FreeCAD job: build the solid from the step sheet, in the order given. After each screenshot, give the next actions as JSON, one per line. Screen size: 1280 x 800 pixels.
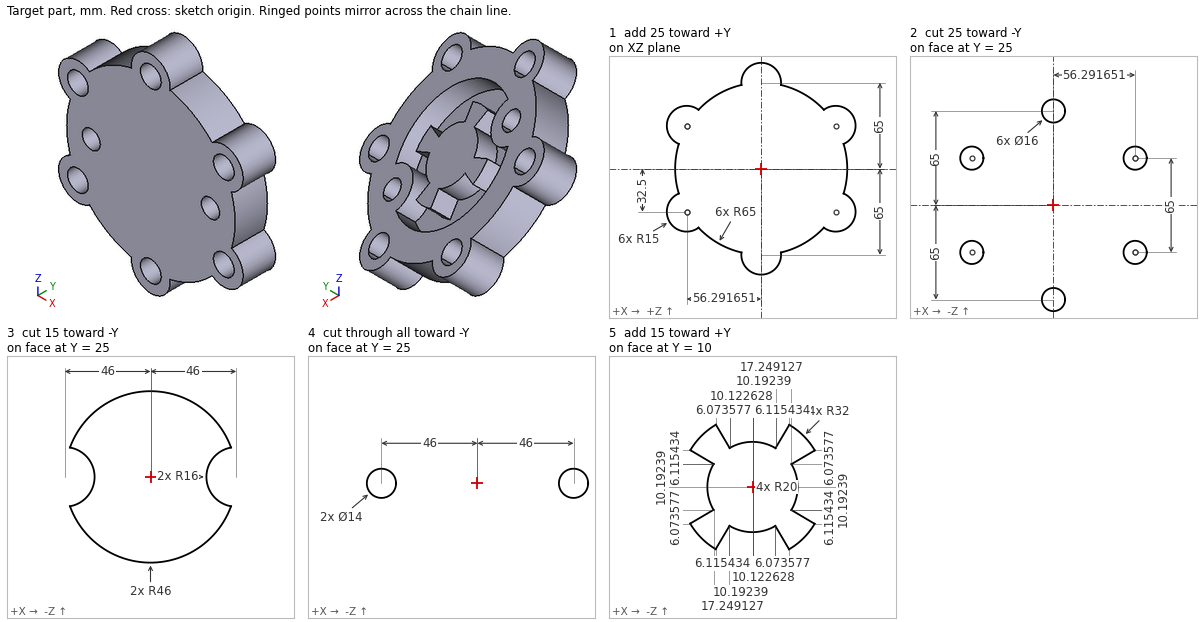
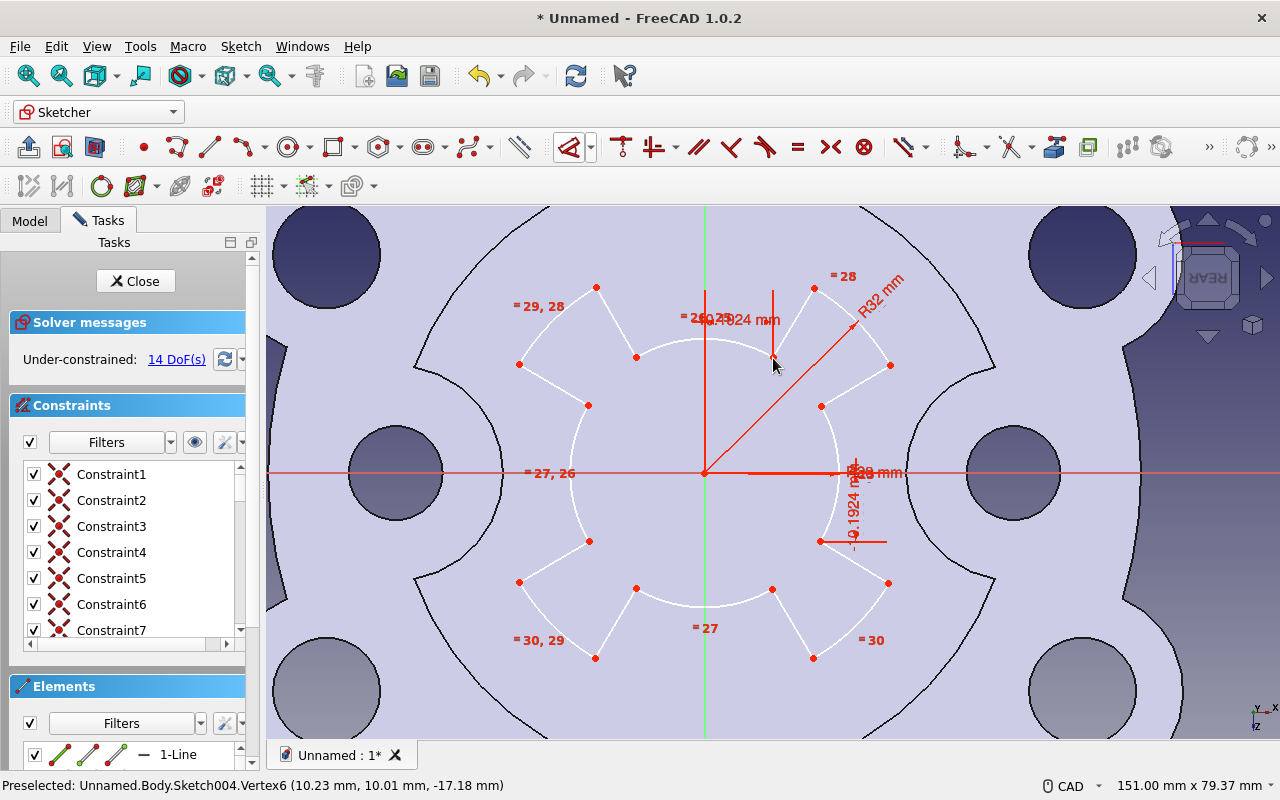
{"action": "left_click", "coordinate": [589, 406]}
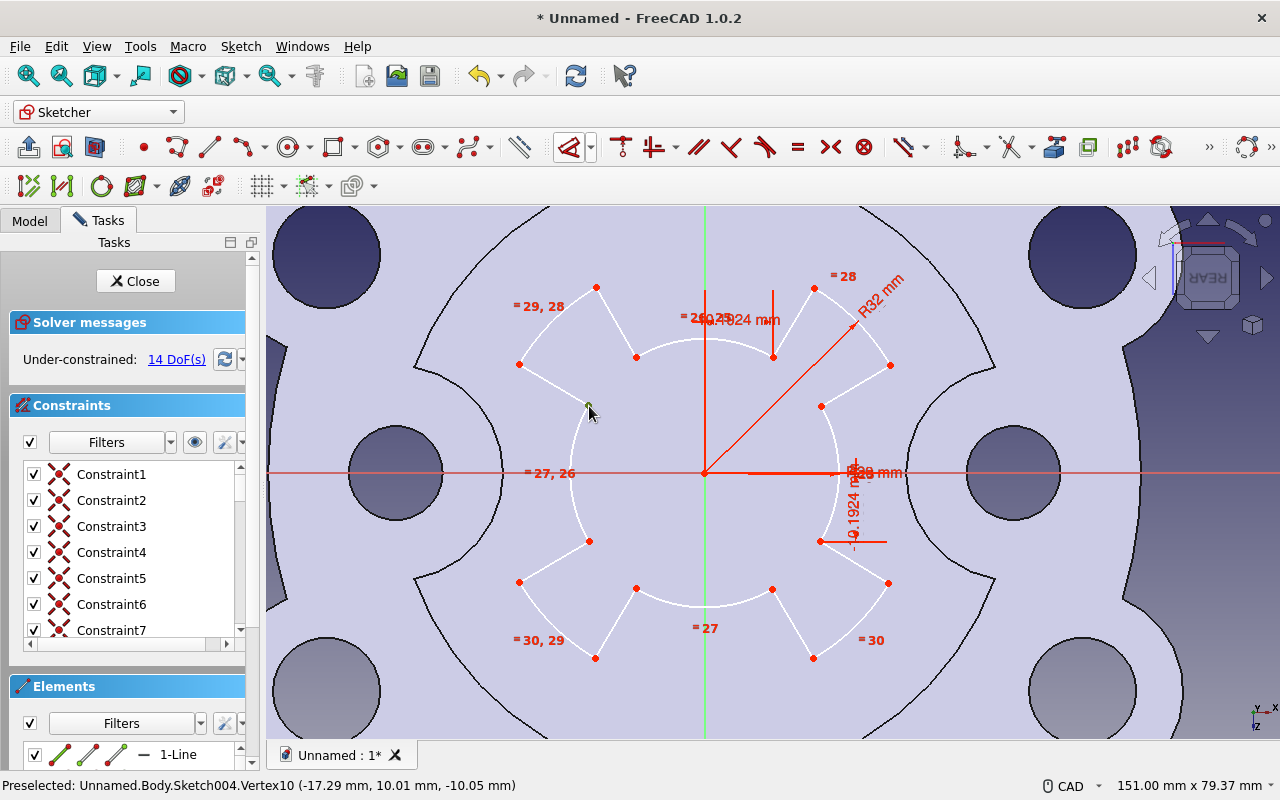
{"action": "left_click", "coordinate": [590, 148]}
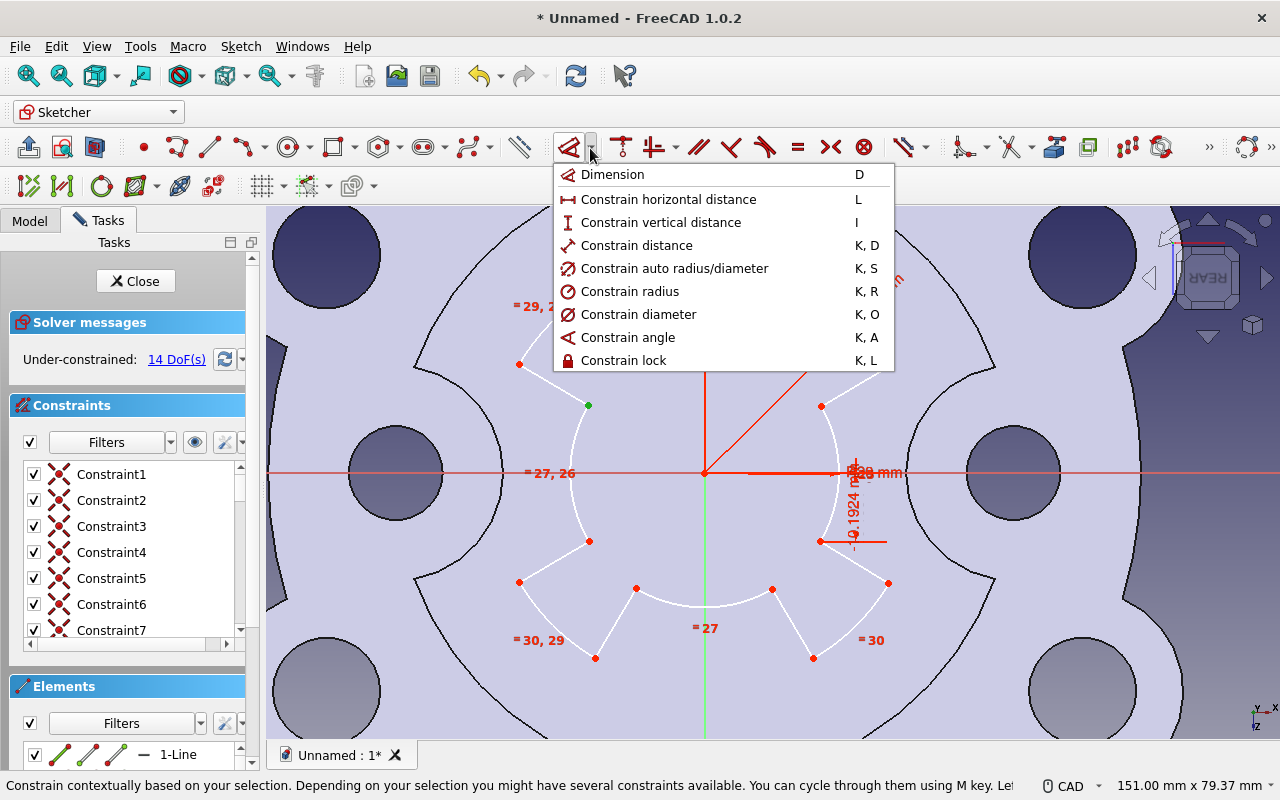
{"action": "left_click", "coordinate": [724, 222]}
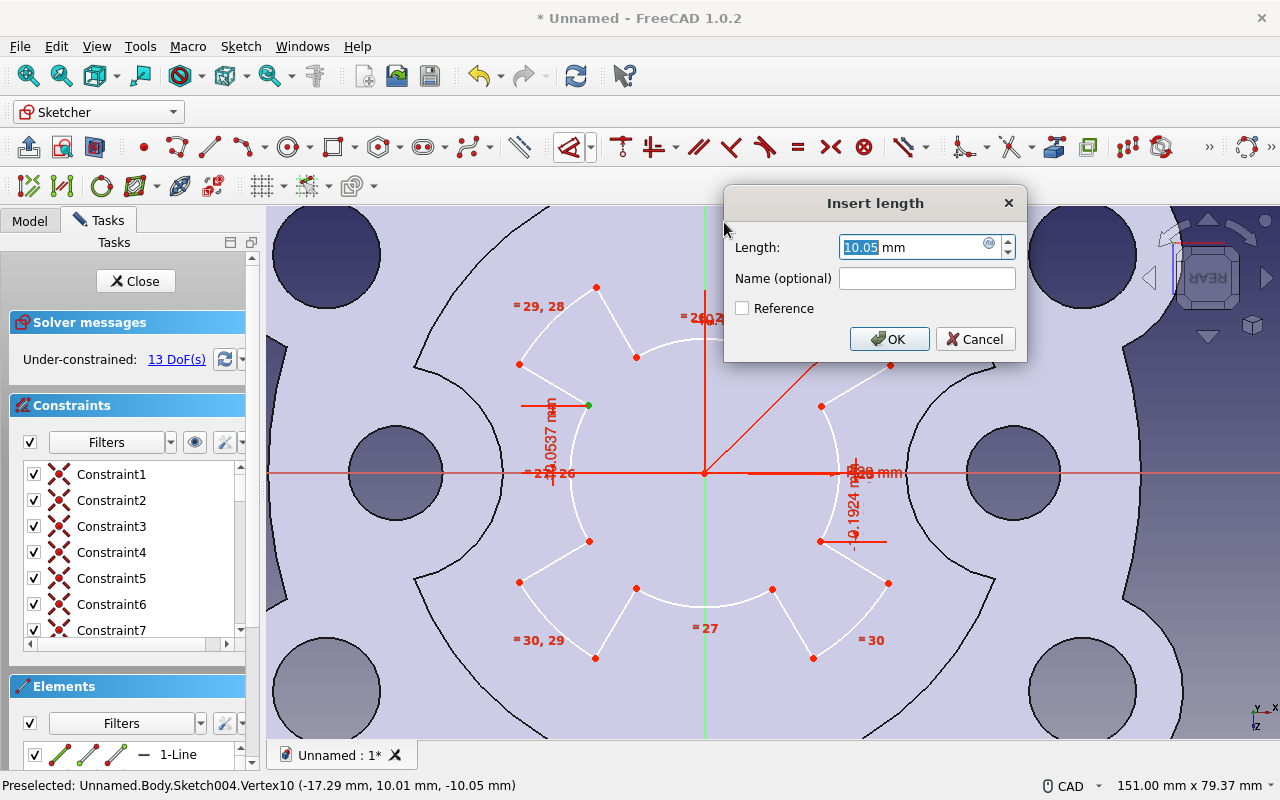
{"action": "type", "text": "10.19239"}
{"action": "key", "text": "Return"}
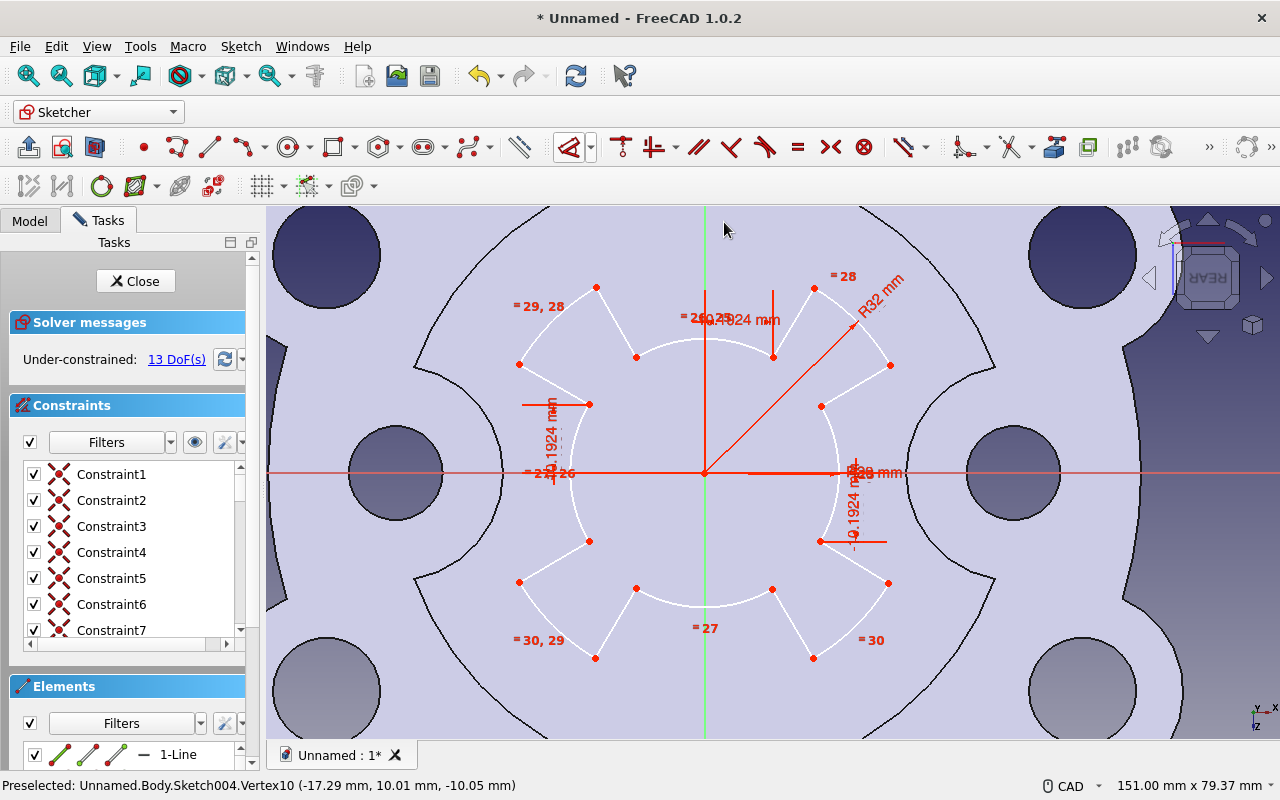
{"action": "left_click", "coordinate": [636, 589]}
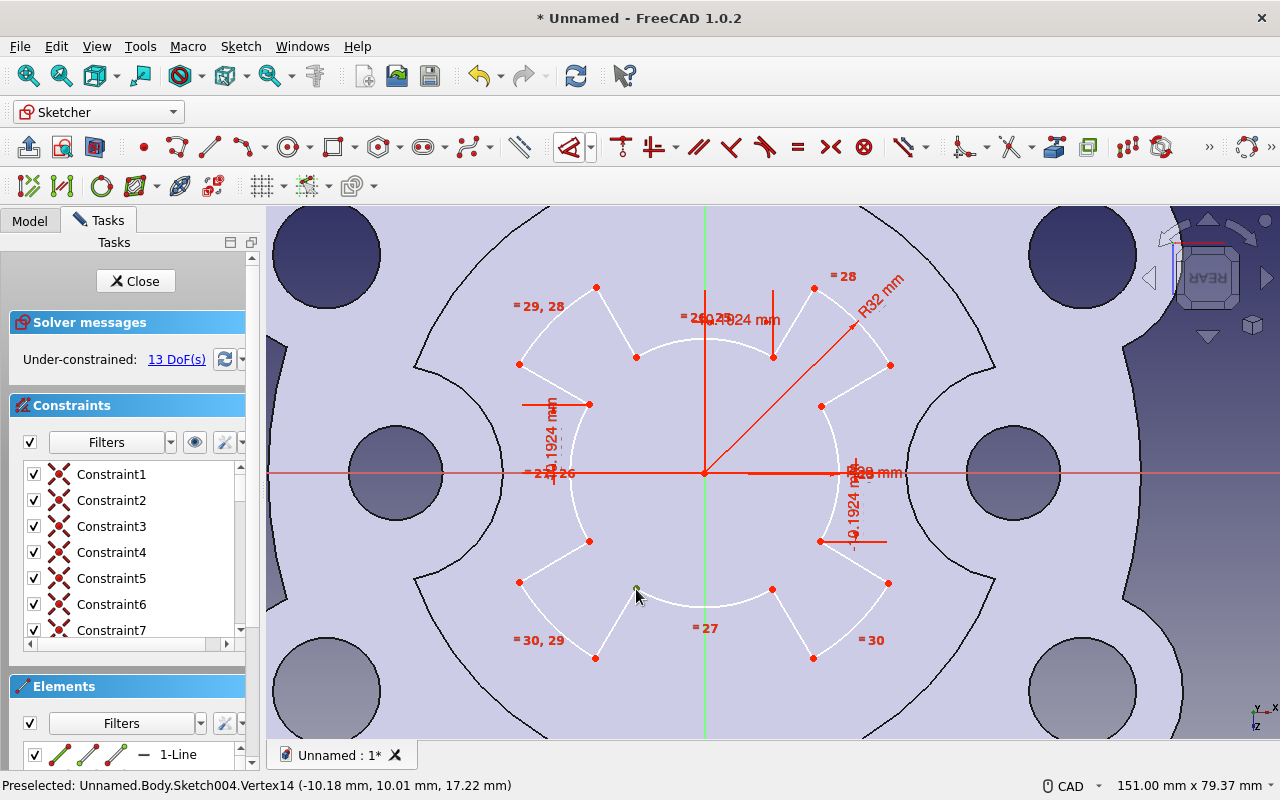
{"action": "left_click", "coordinate": [590, 148]}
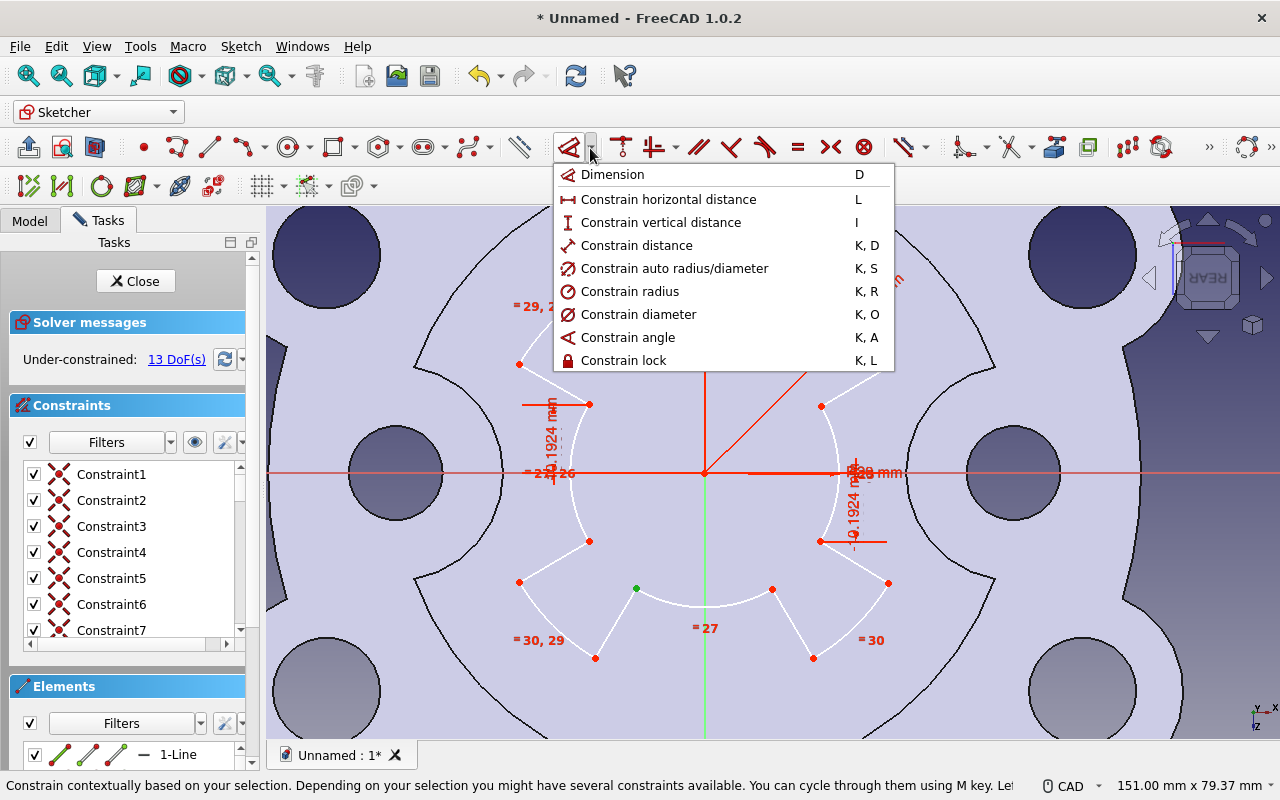
{"action": "left_click", "coordinate": [724, 200]}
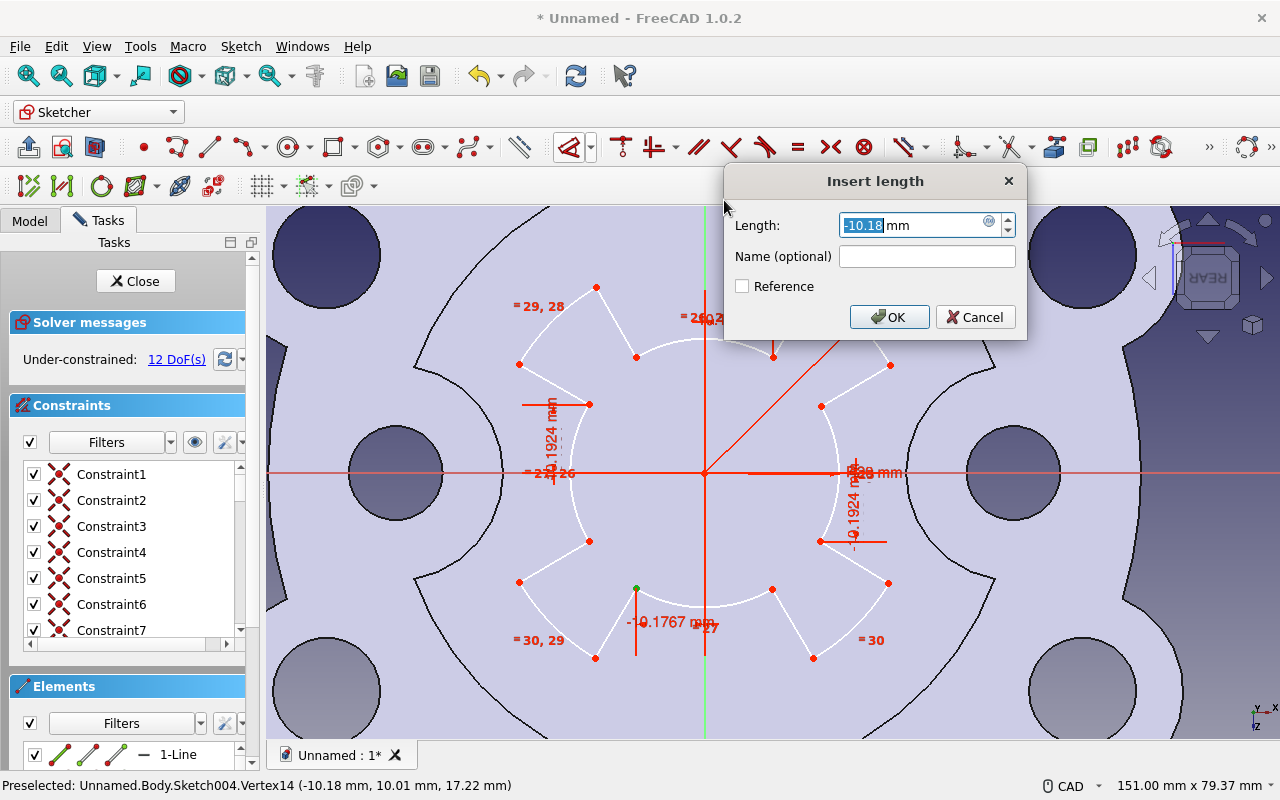
{"action": "type", "text": "-10.19239"}
{"action": "key", "text": "Return"}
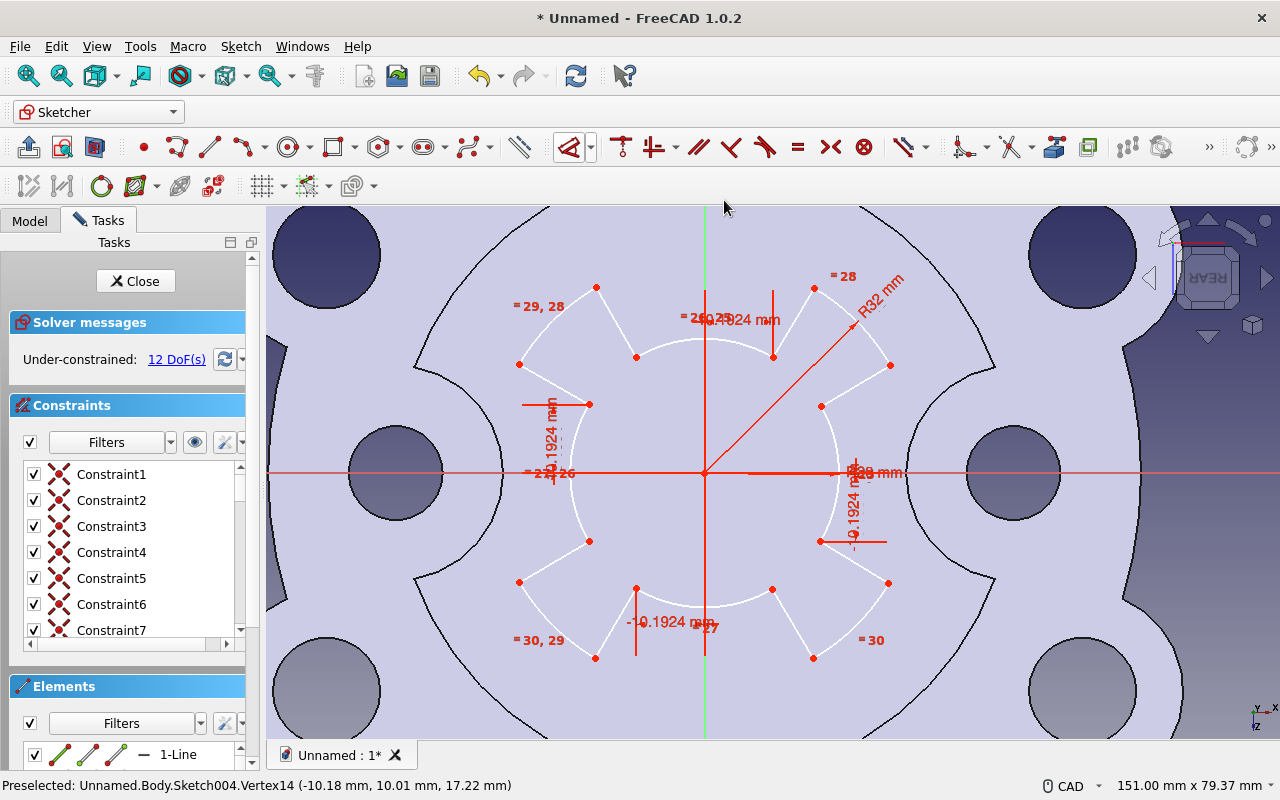
{"action": "left_click", "coordinate": [868, 571]}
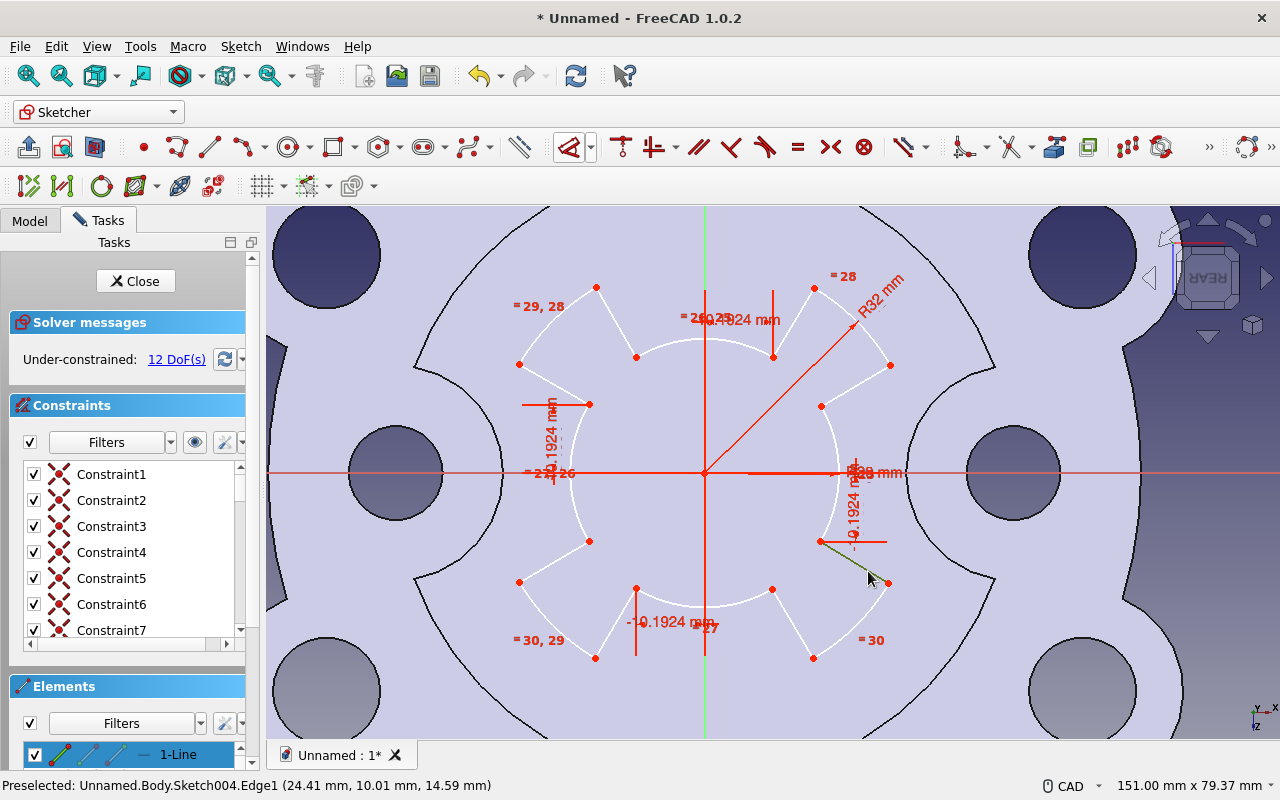
{"action": "left_click", "coordinate": [590, 148]}